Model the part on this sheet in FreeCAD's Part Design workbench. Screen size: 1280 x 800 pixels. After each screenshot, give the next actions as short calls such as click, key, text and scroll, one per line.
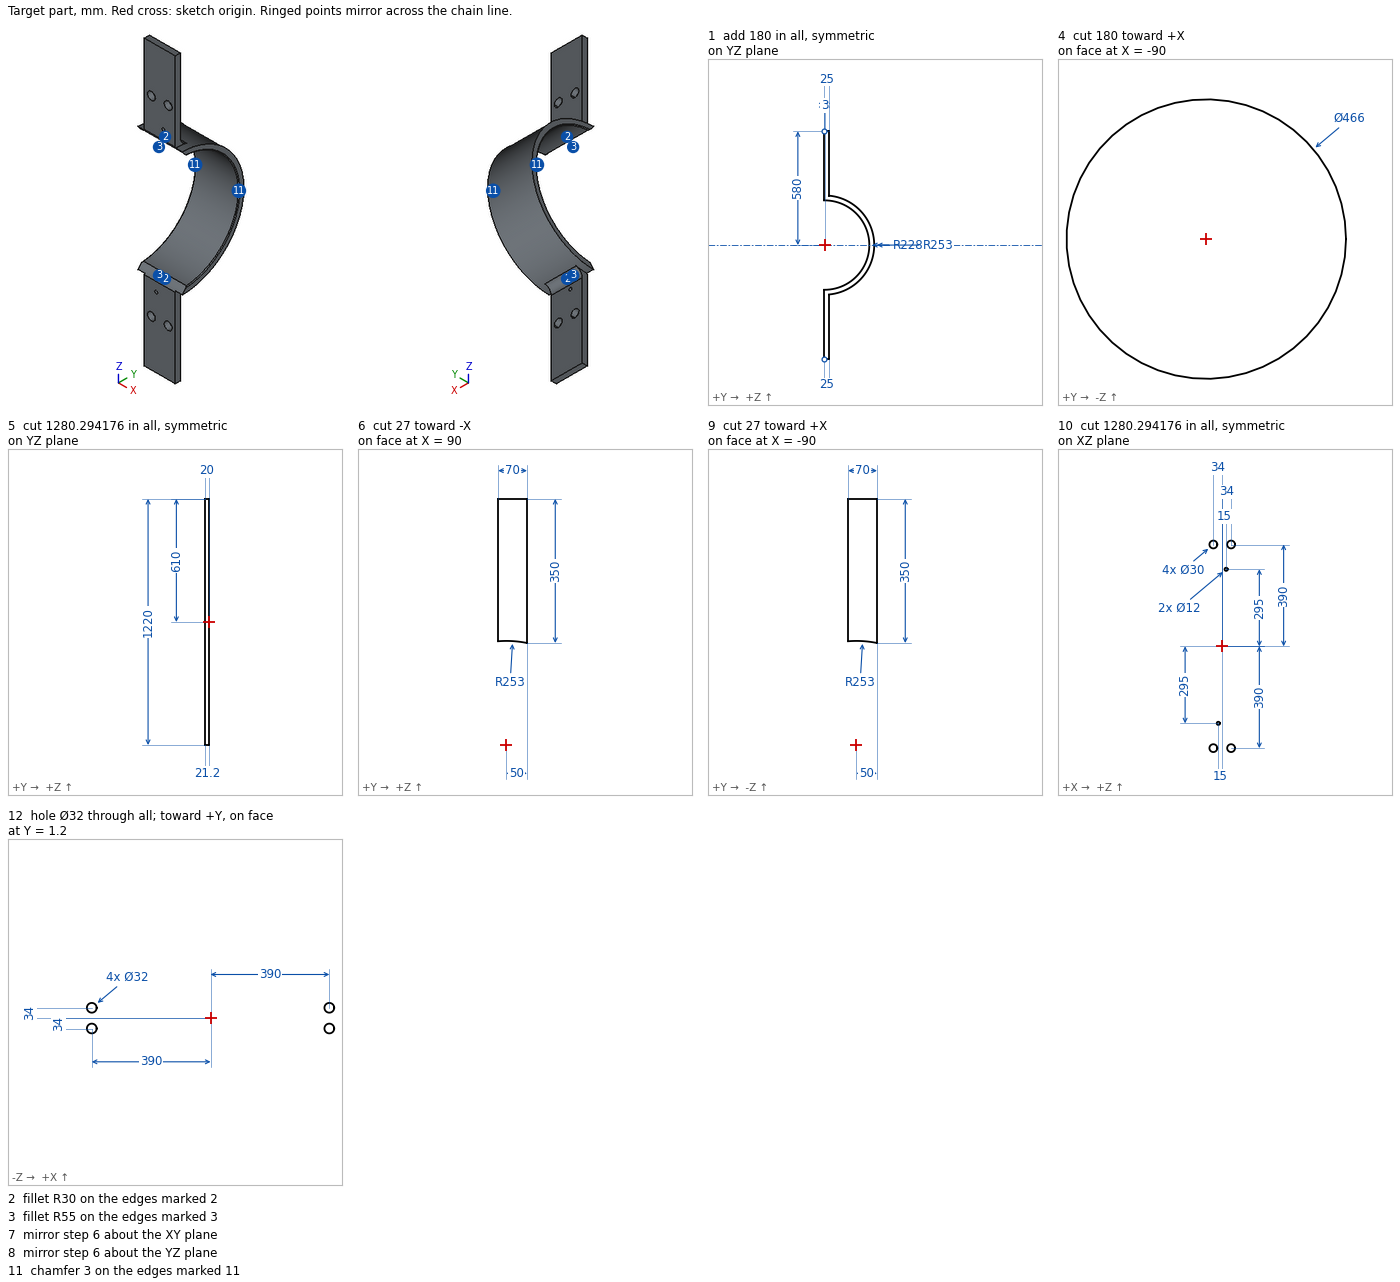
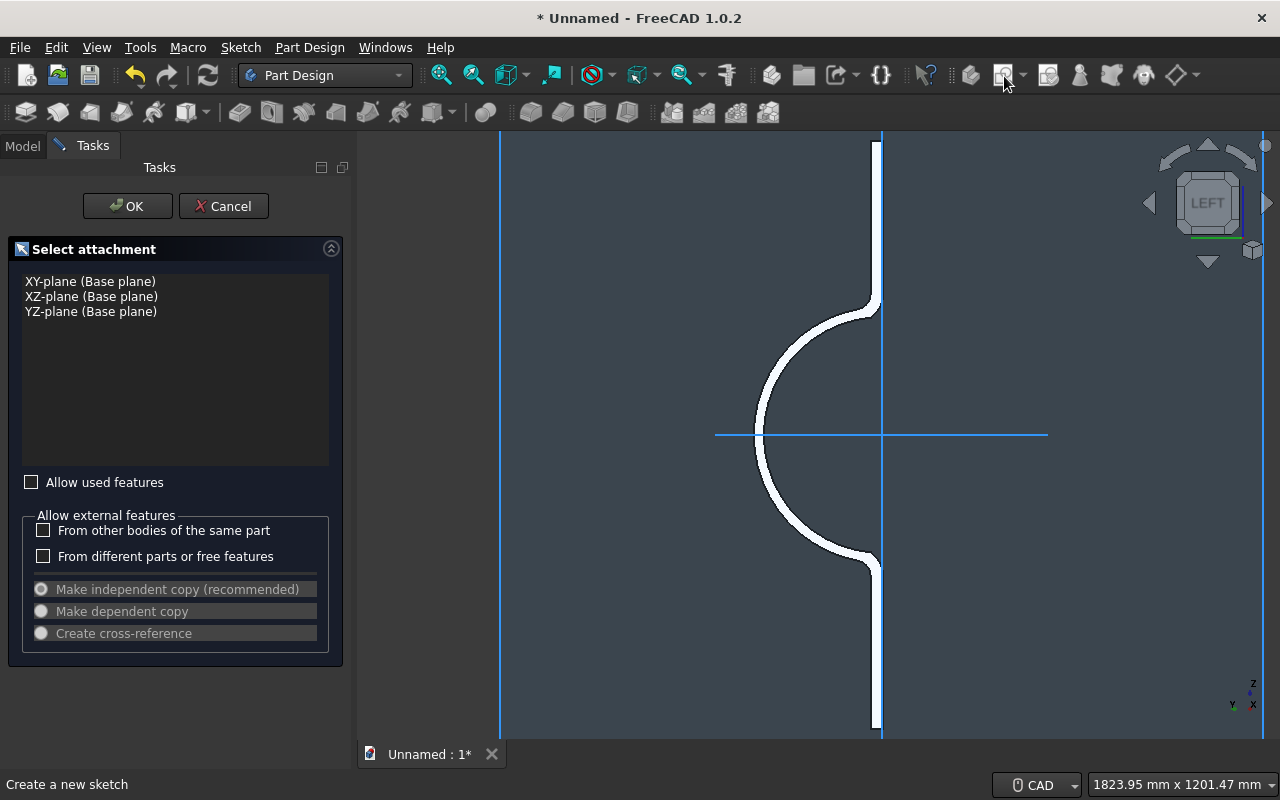
click(82, 312)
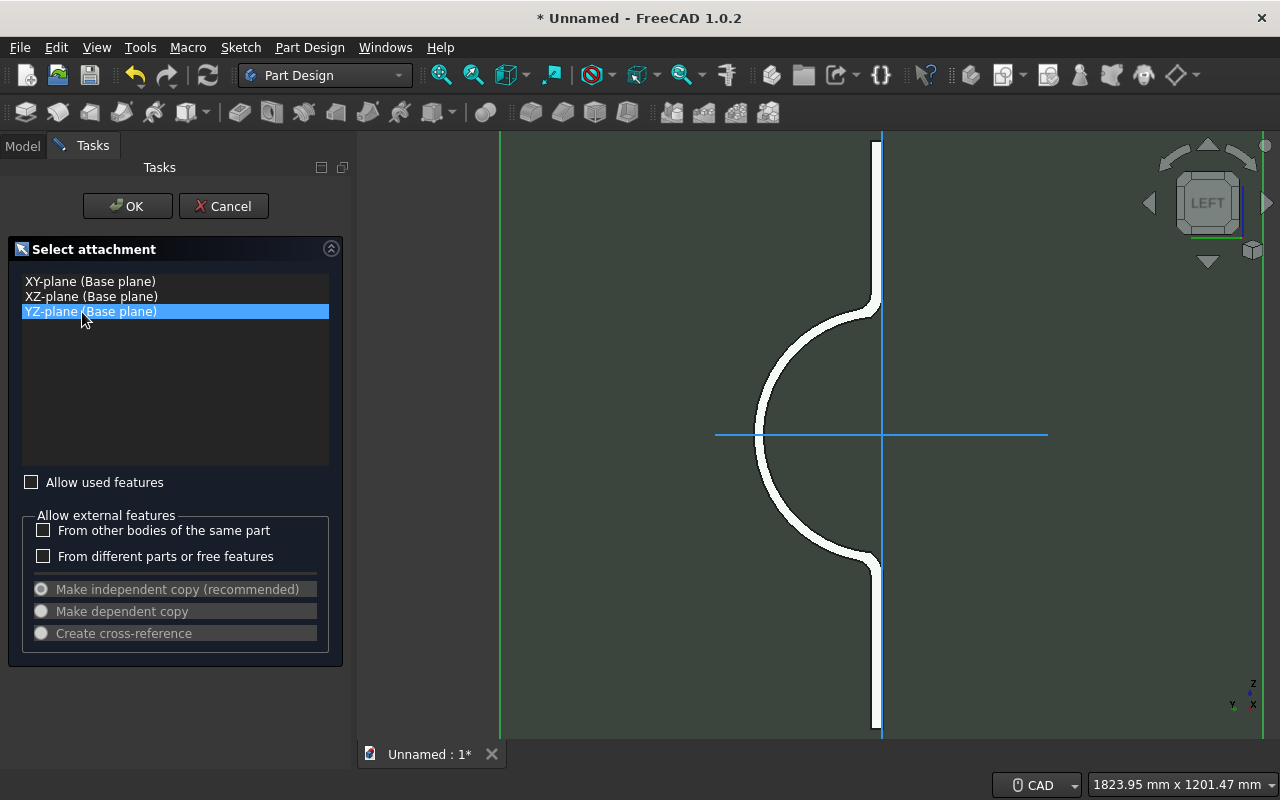
click(128, 206)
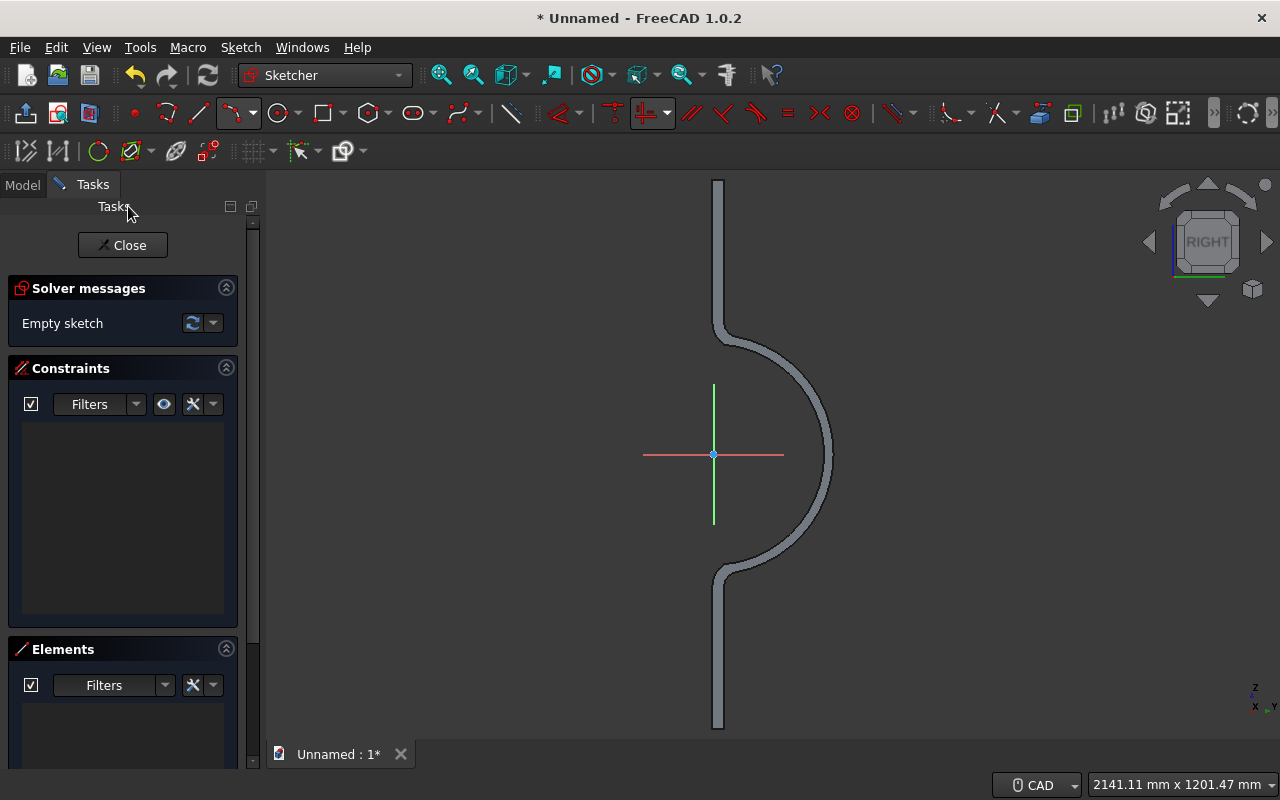
click(90, 114)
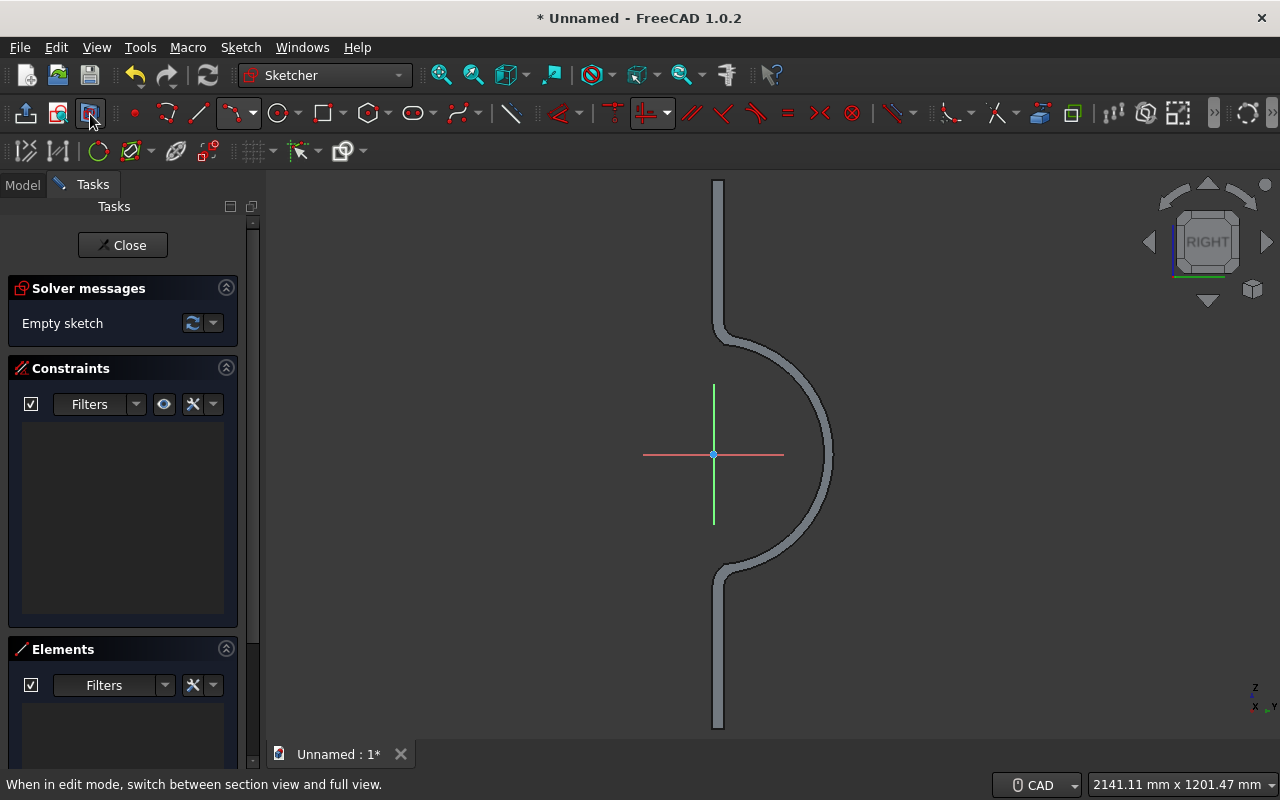
scroll(695, 455, down, 2)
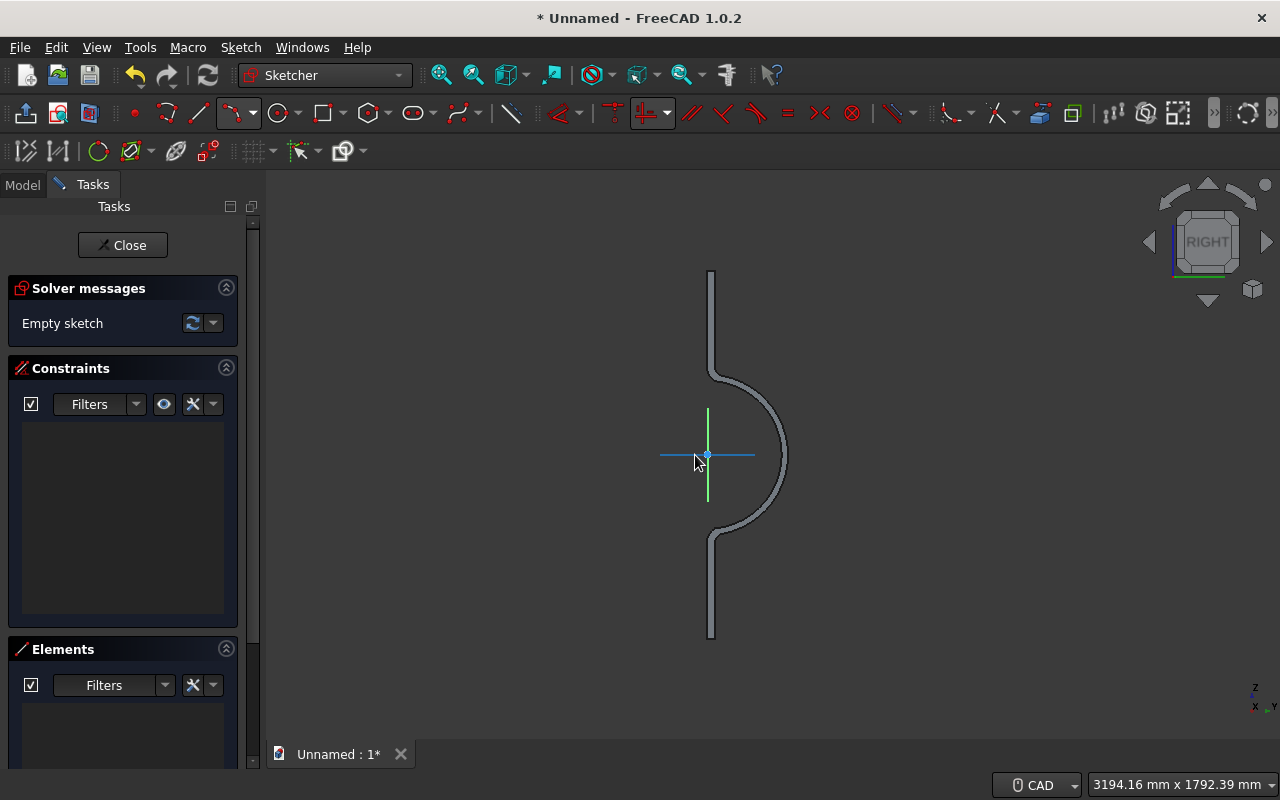
click(324, 114)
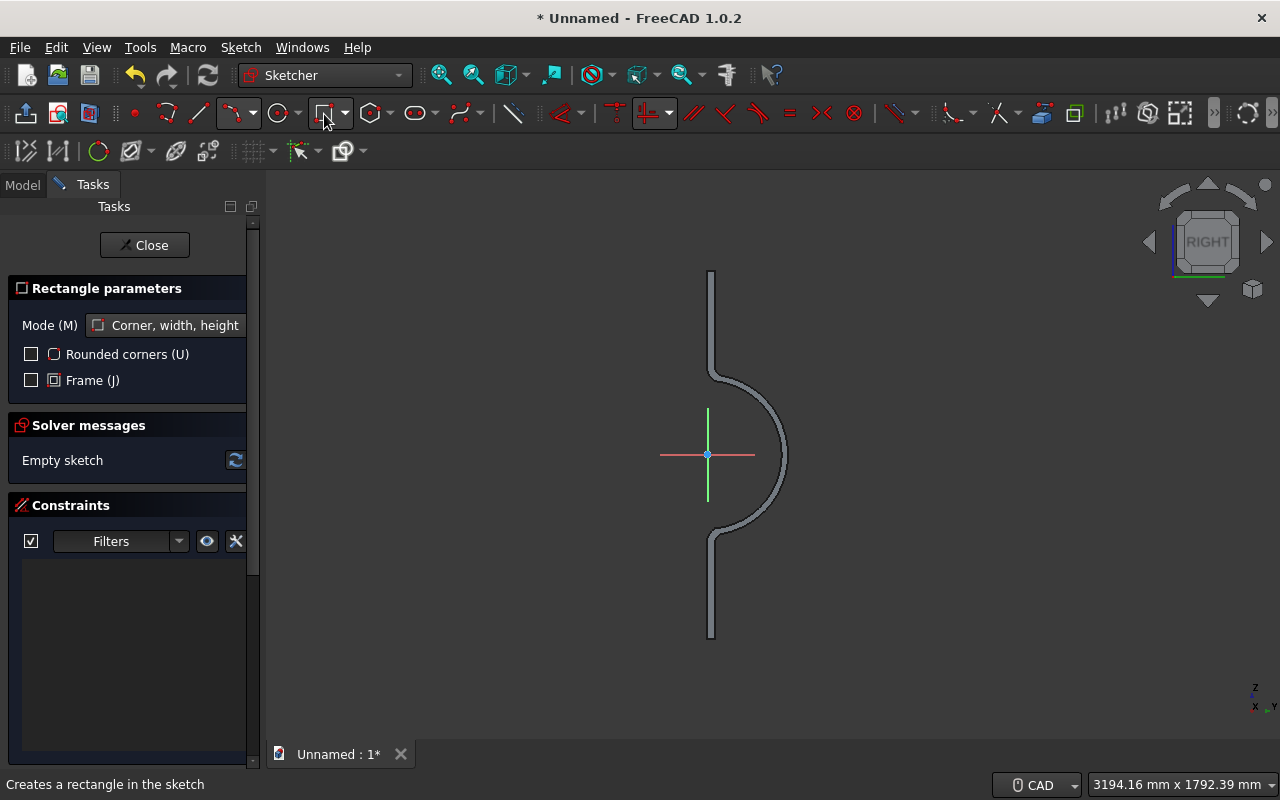
scroll(701, 261, up, 5)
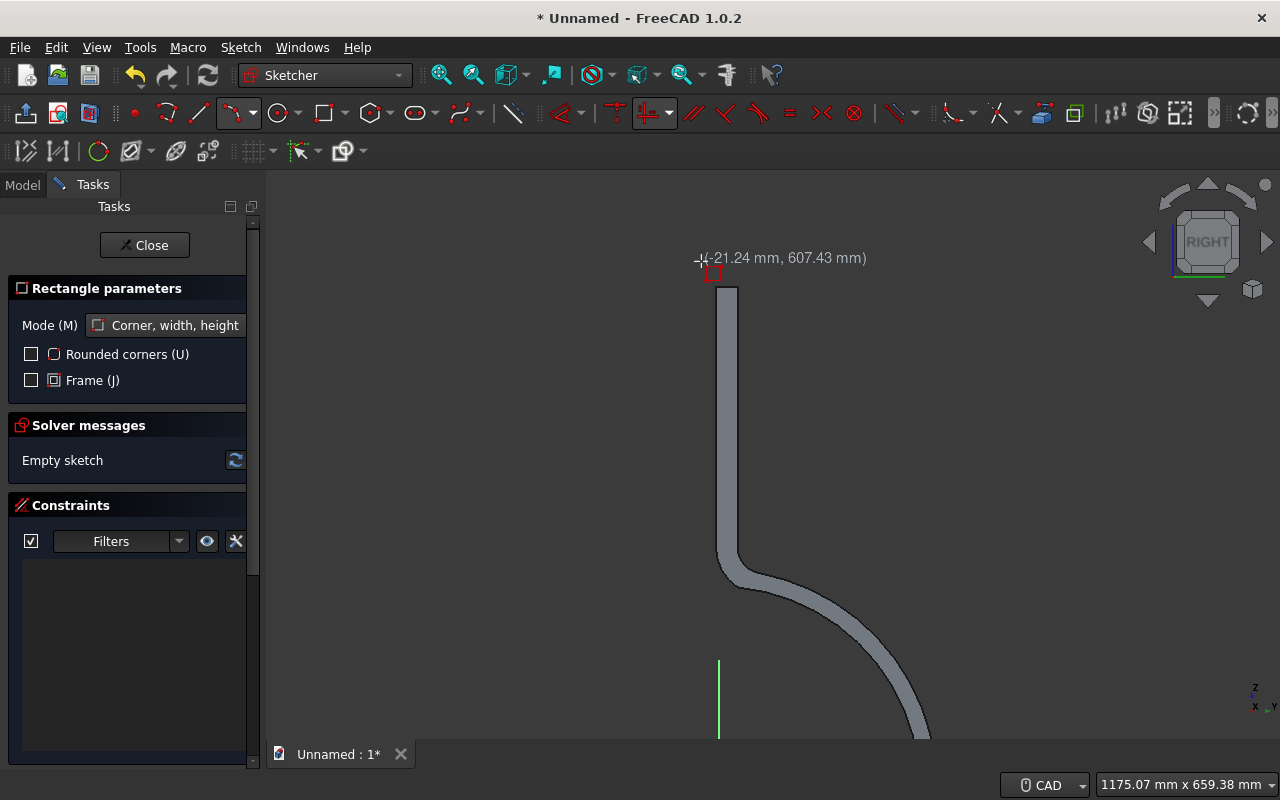
click(701, 261)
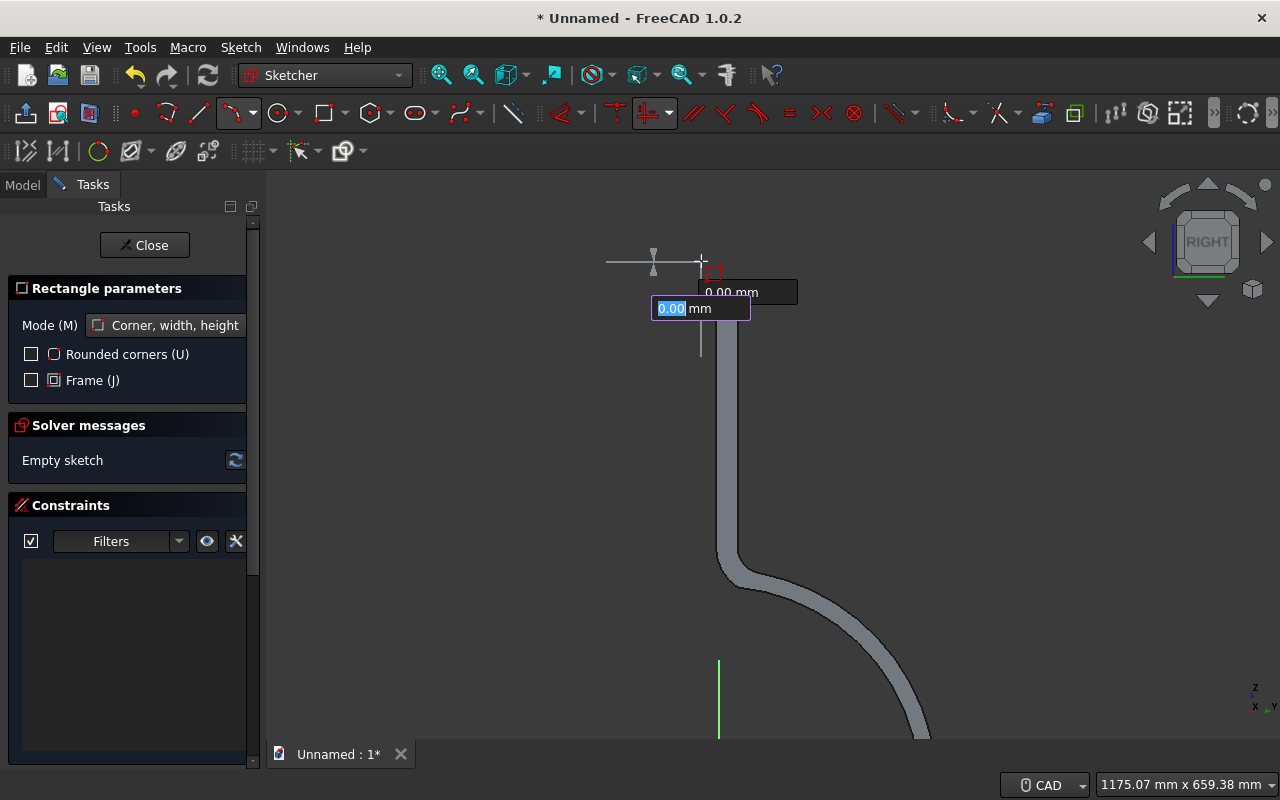
scroll(701, 261, down, 5)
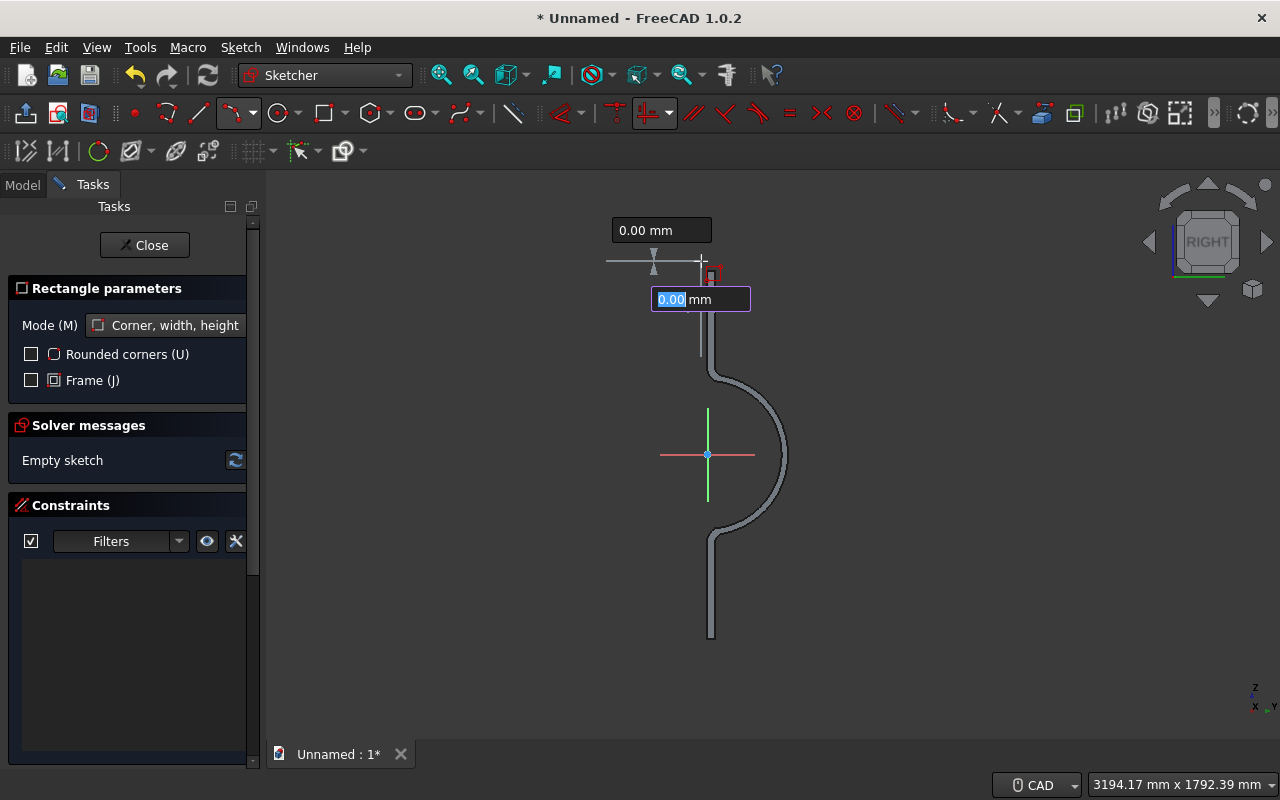
scroll(708, 648, up, 19)